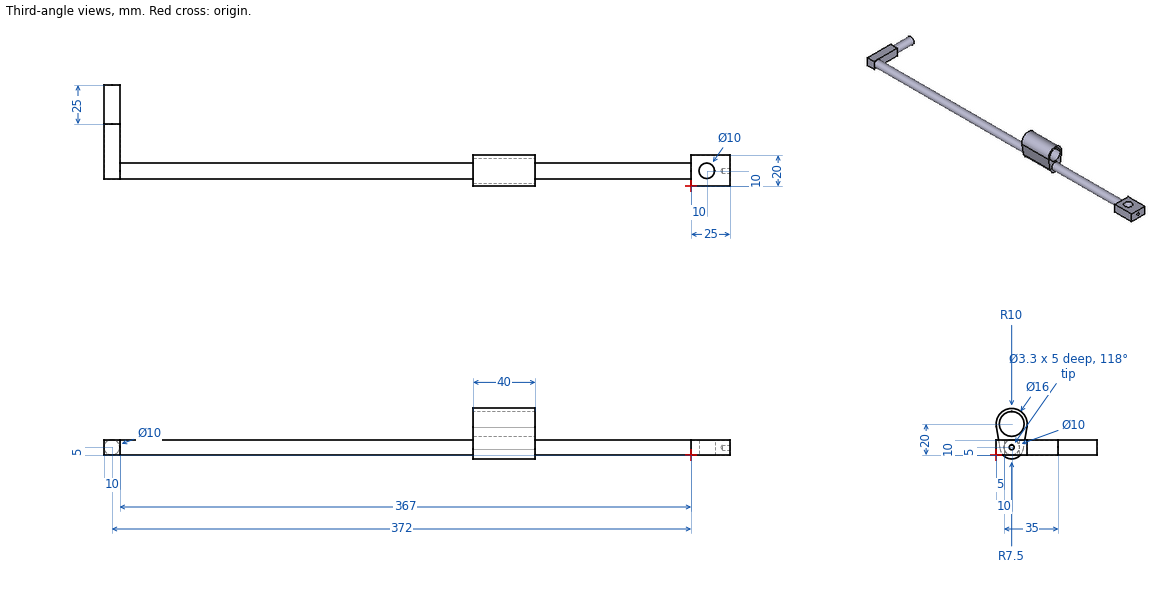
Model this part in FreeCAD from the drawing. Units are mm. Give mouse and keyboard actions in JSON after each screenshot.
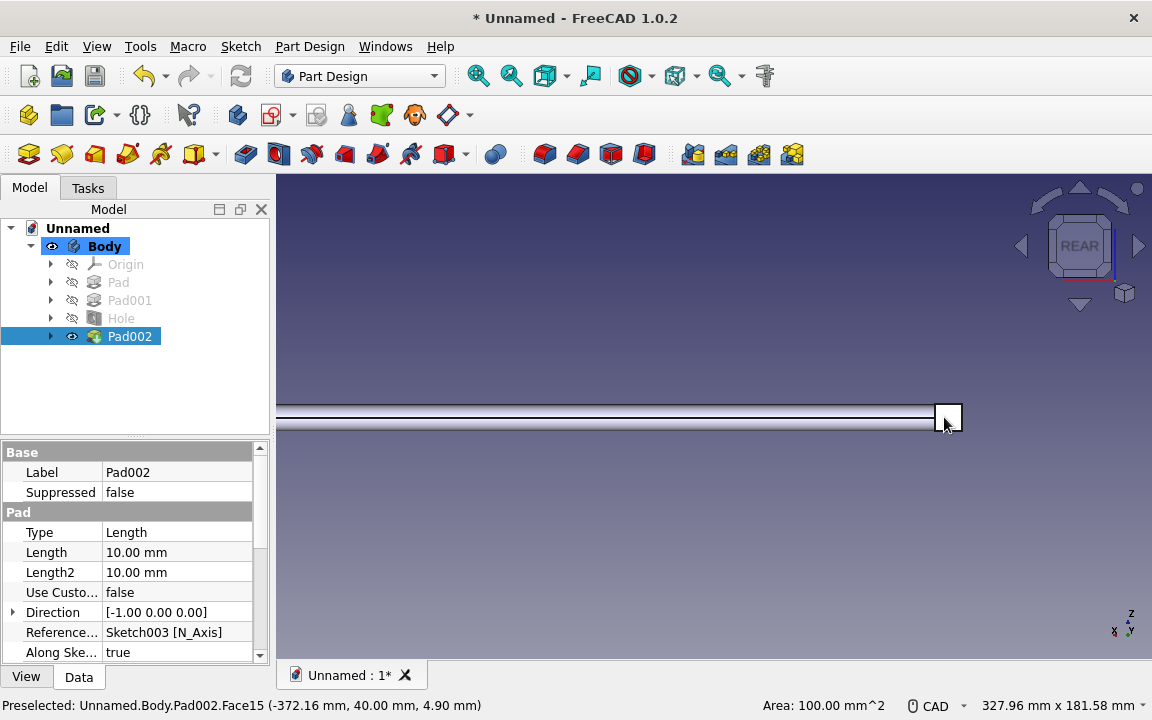
{"action": "left_click", "coordinate": [270, 116]}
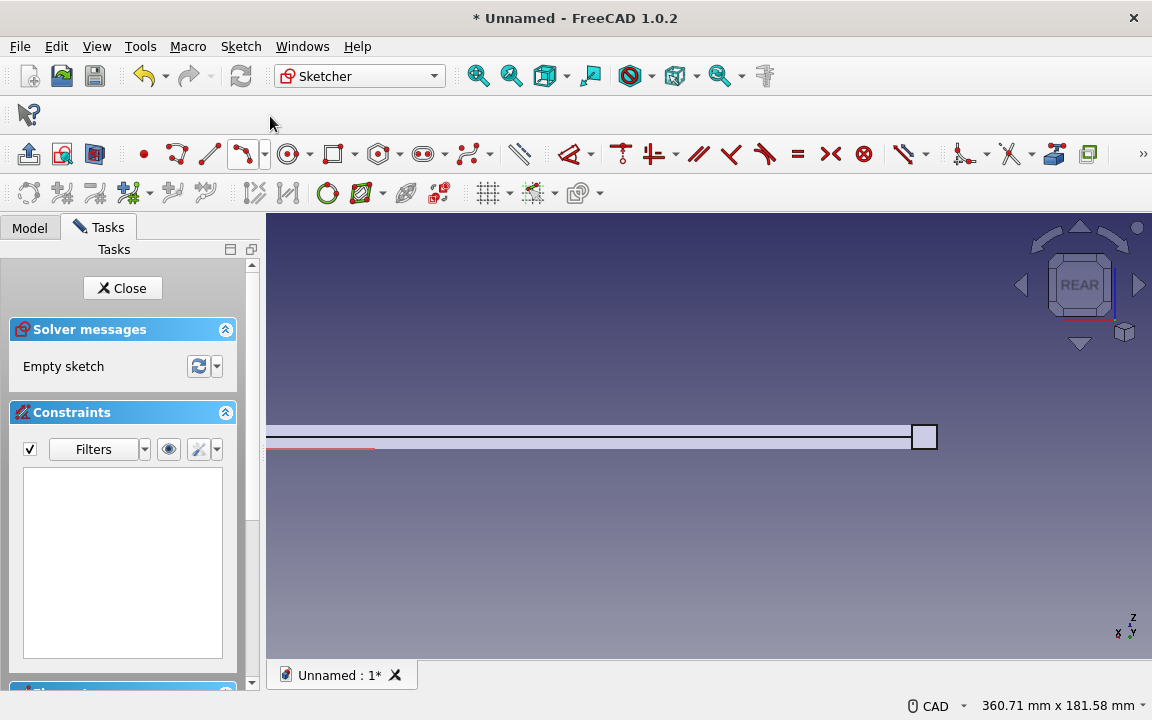
{"action": "scroll", "coordinate": [953, 437], "scroll_direction": "up", "scroll_amount": 12}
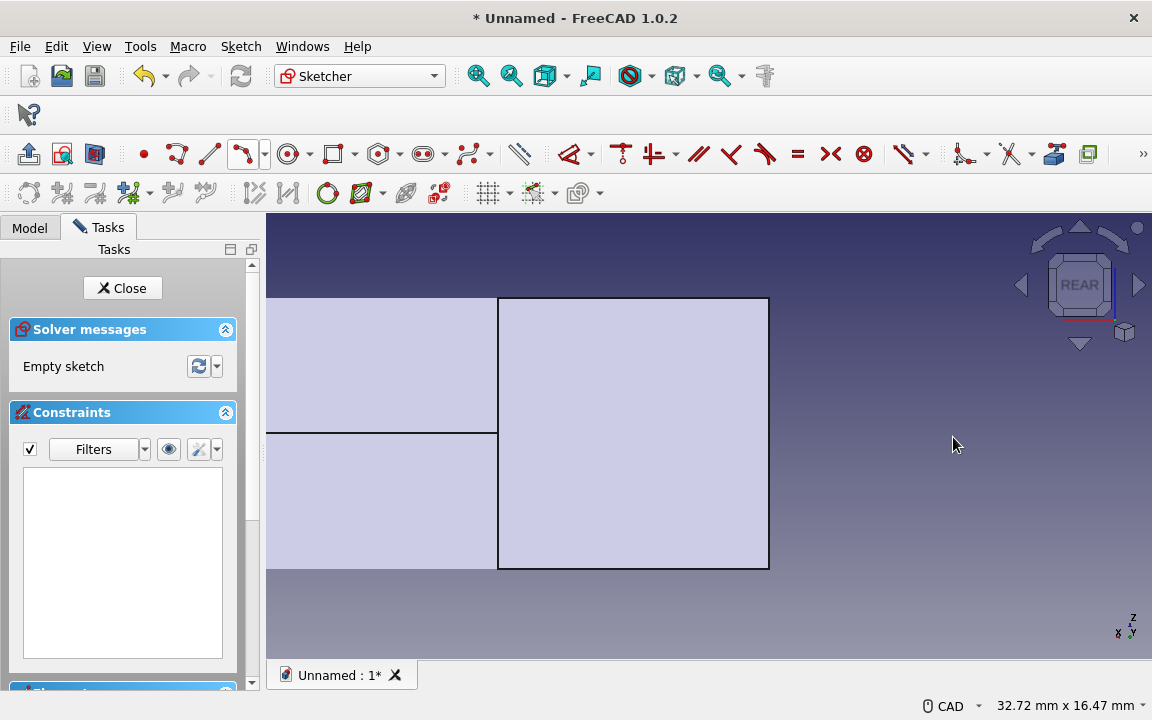
{"action": "key", "text": "g c"}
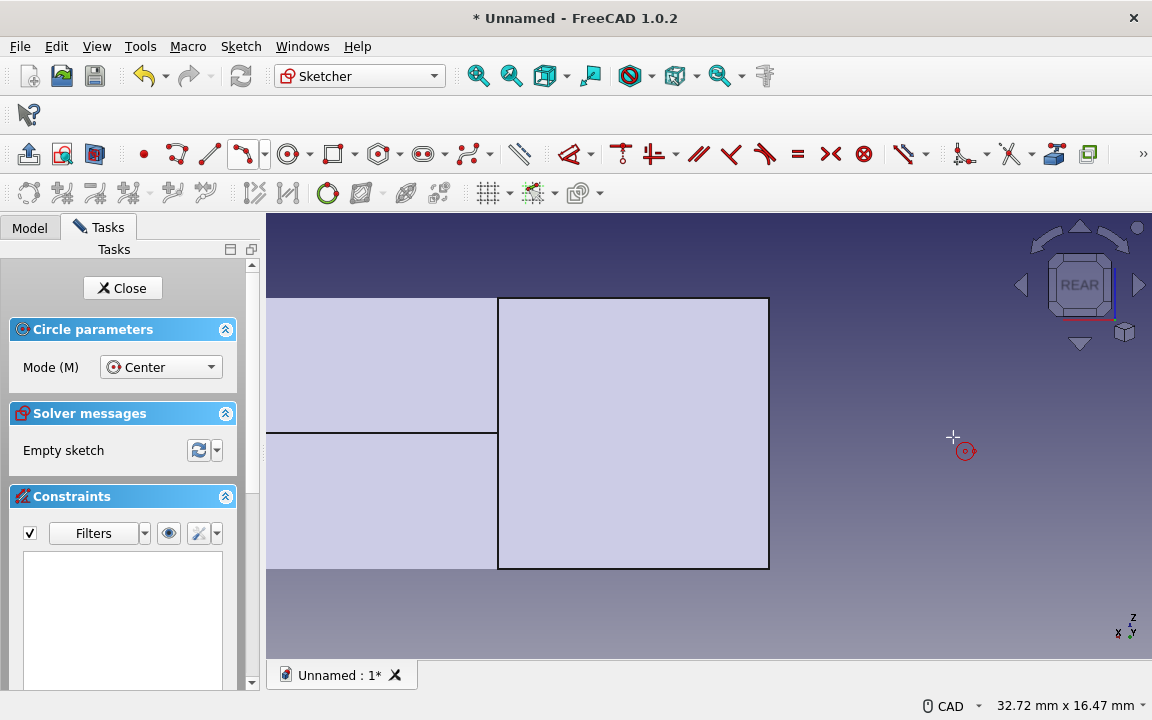
{"action": "left_click", "coordinate": [633, 433]}
{"action": "mouse_move", "coordinate": [729, 338]}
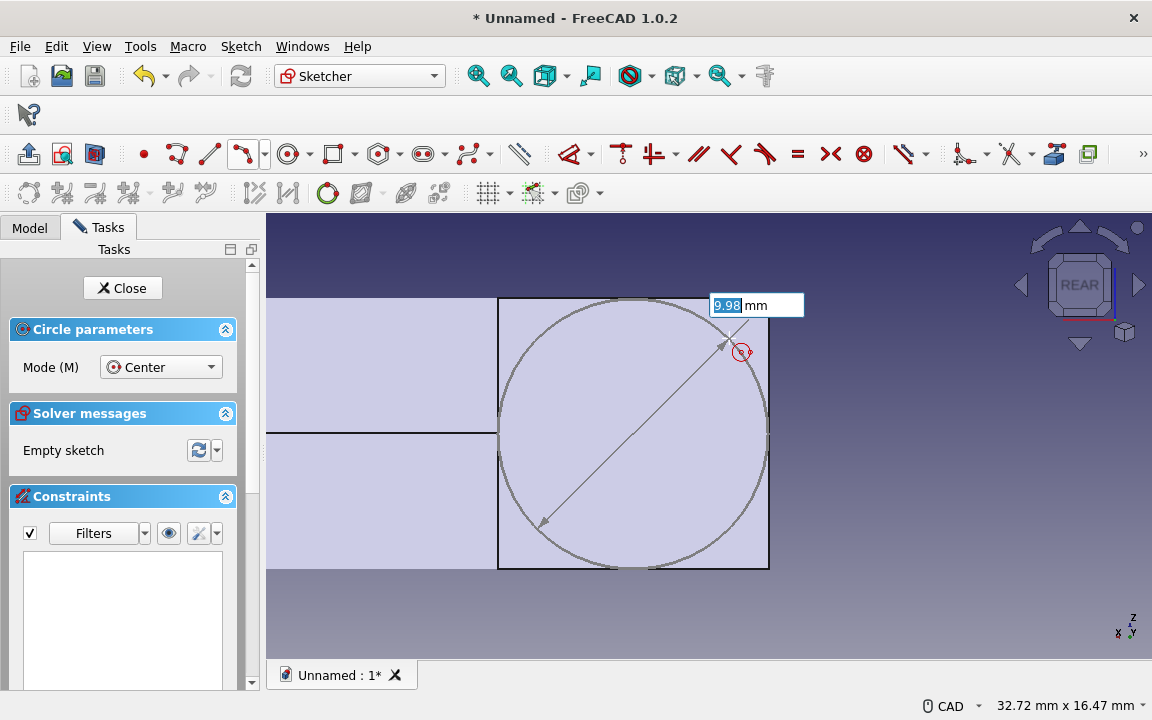
{"action": "type", "text": "10"}
{"action": "key", "text": "Return"}
{"action": "key", "text": "Escape"}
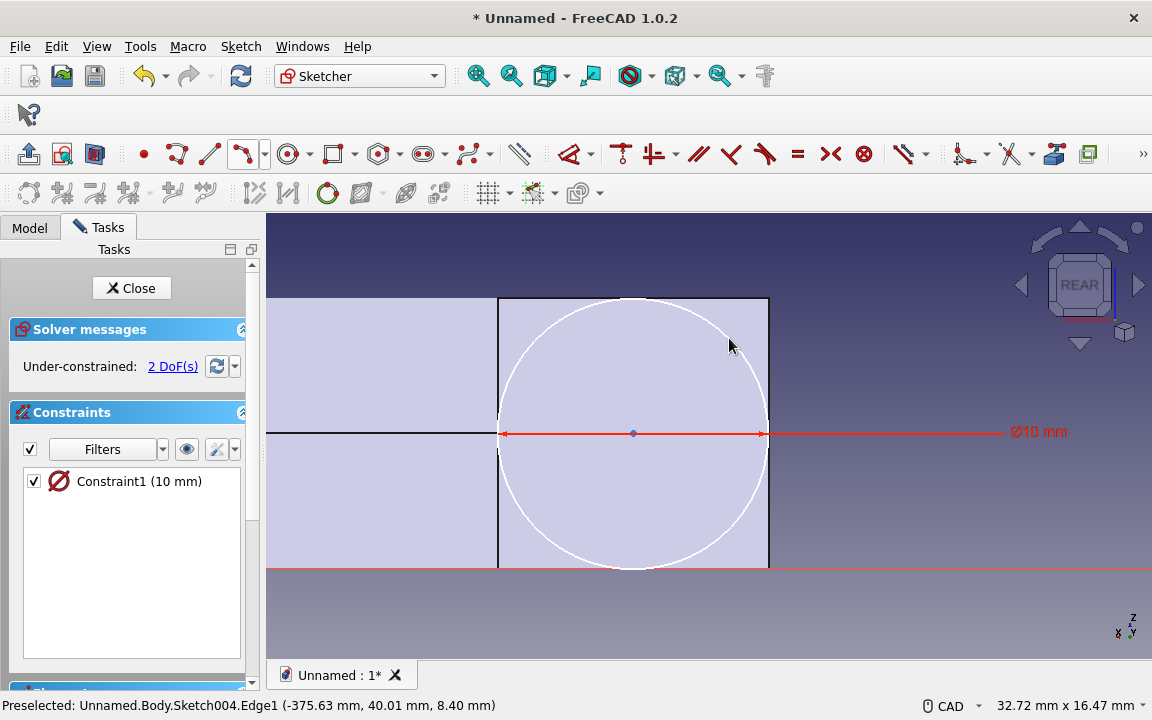
{"action": "key", "text": "d"}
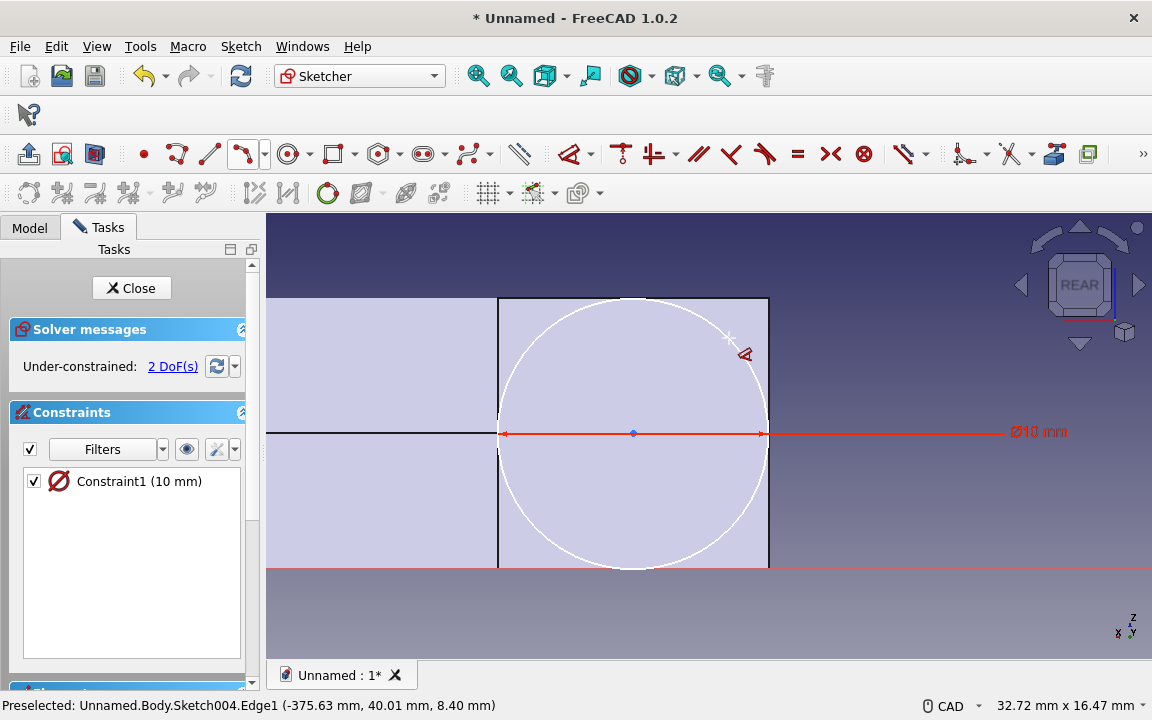
{"action": "left_click", "coordinate": [633, 434]}
{"action": "left_click", "coordinate": [667, 501]}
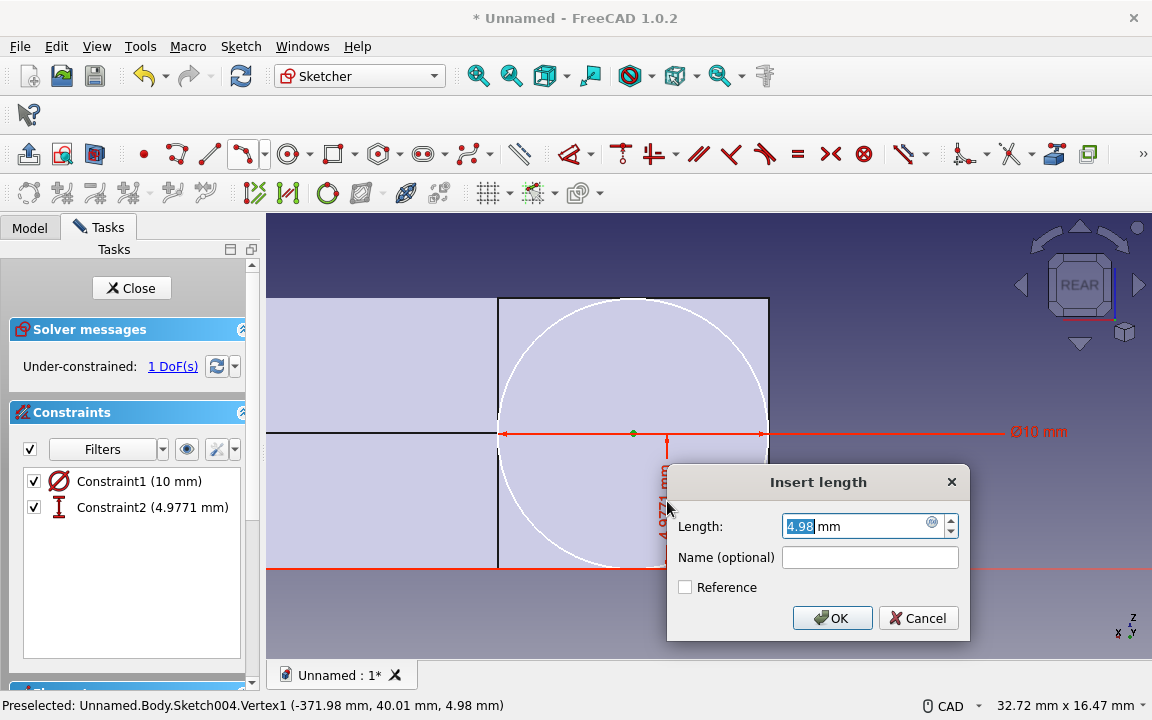
{"action": "type", "text": "5"}
{"action": "key", "text": "Return"}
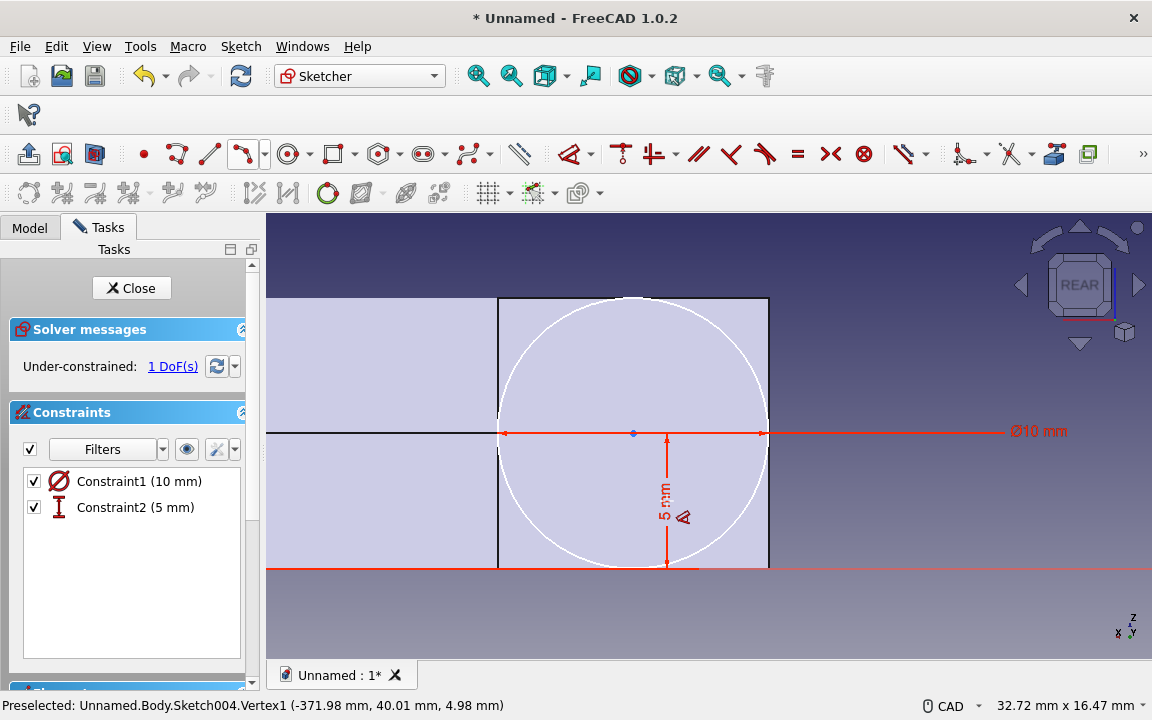
{"action": "left_click", "coordinate": [633, 433]}
{"action": "left_click", "coordinate": [464, 603]}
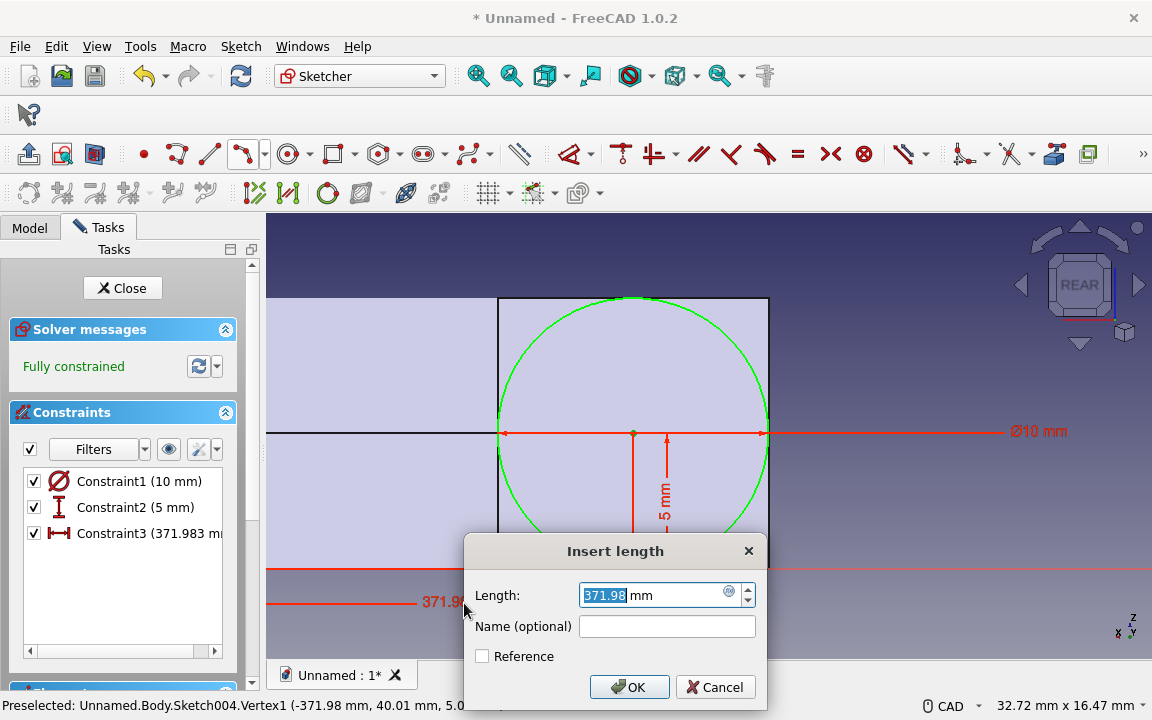
{"action": "type", "text": "372"}
{"action": "key", "text": "Return"}
{"action": "key", "text": "Escape"}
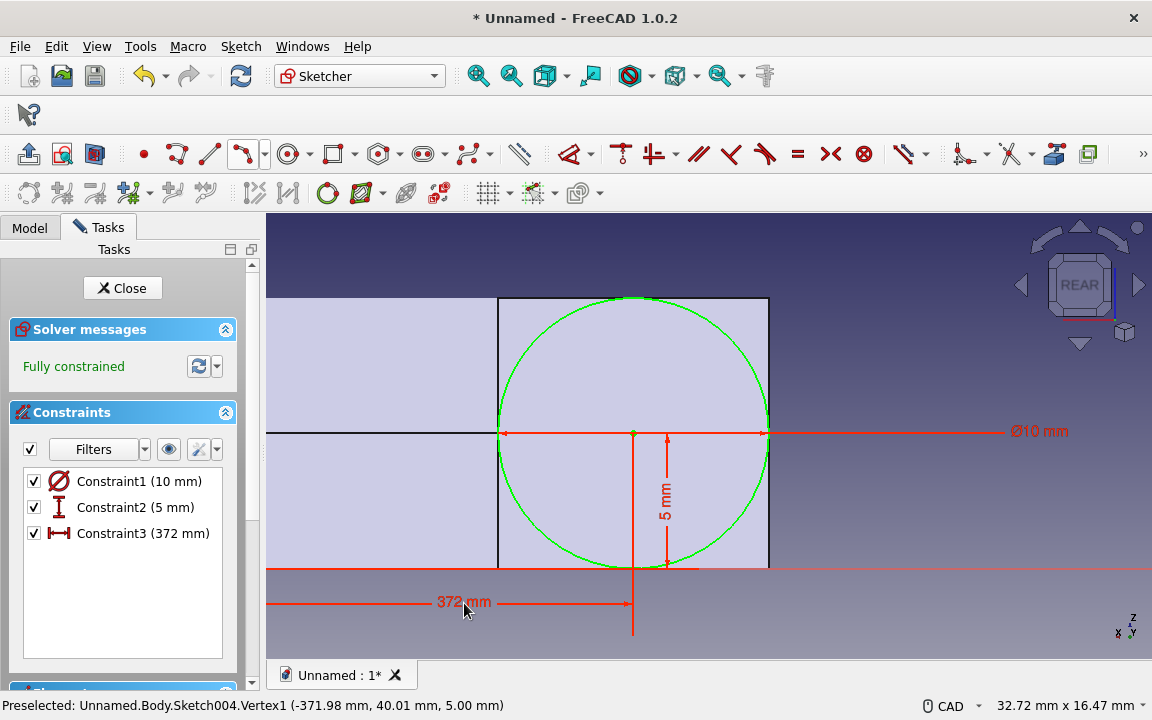
{"action": "left_click", "coordinate": [123, 288]}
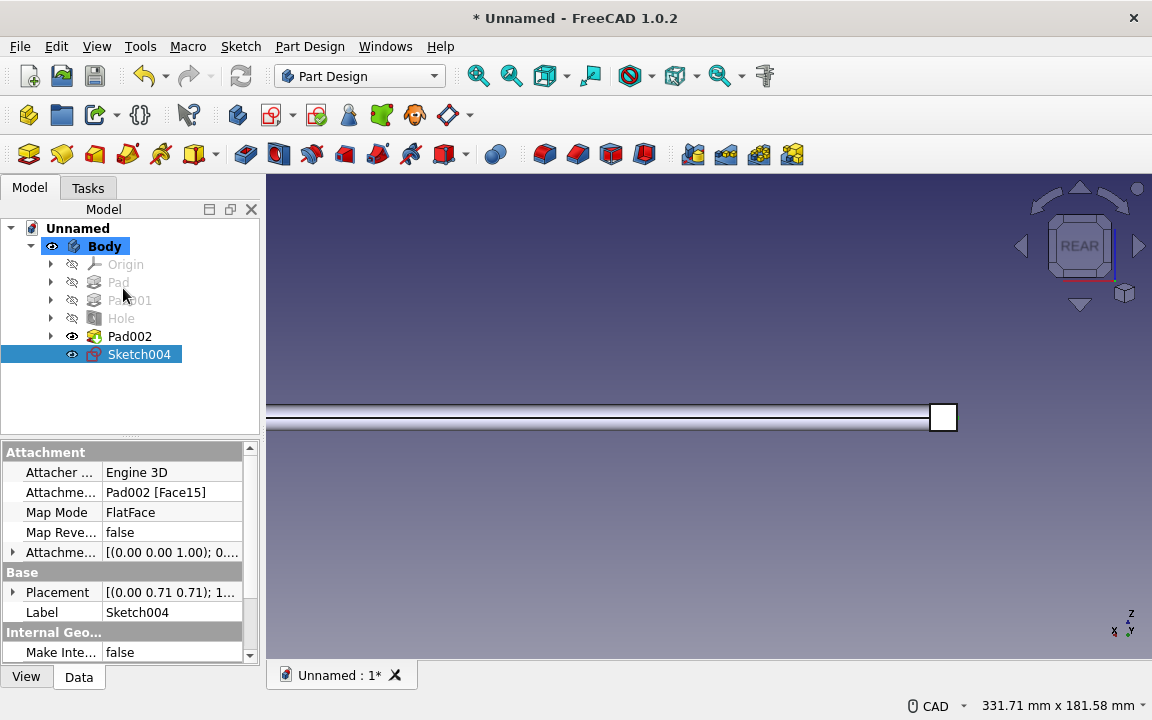
{"action": "left_click", "coordinate": [29, 154]}